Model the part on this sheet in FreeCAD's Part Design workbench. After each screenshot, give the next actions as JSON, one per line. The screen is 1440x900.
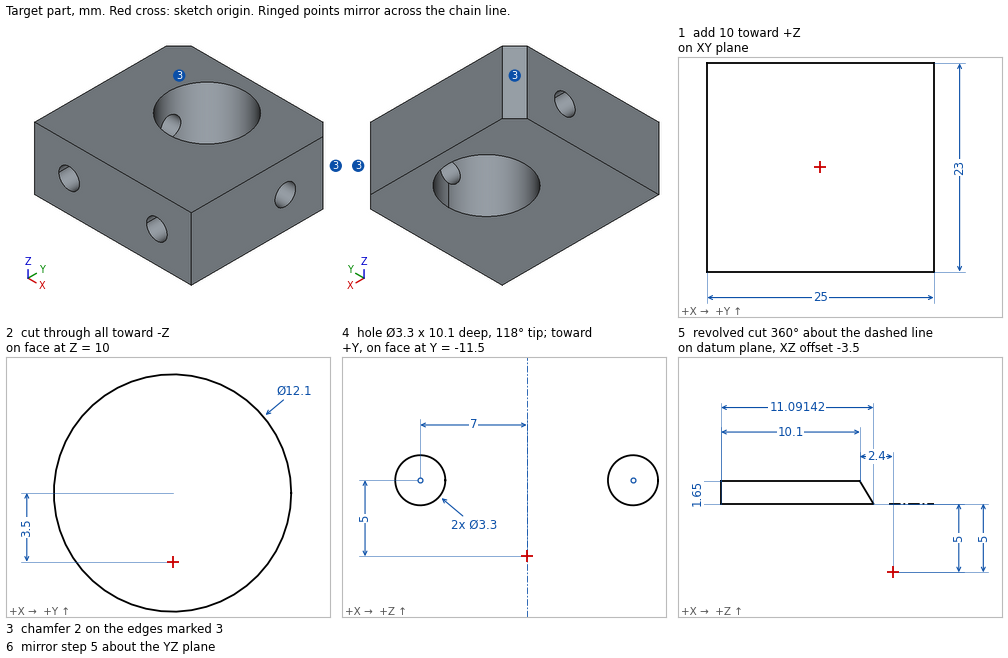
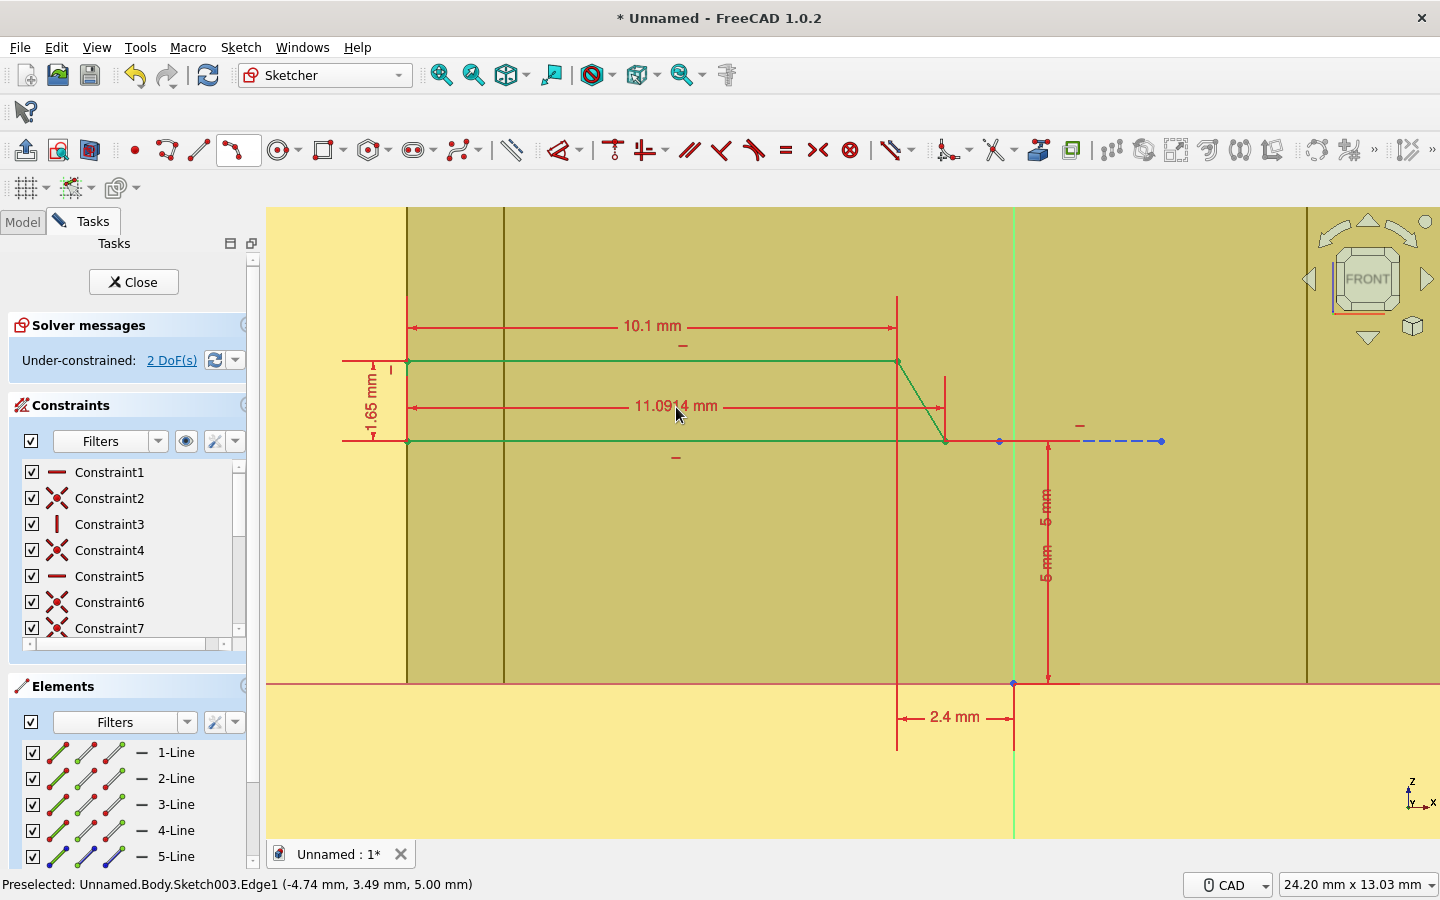
{"action": "left_click", "coordinate": [134, 282]}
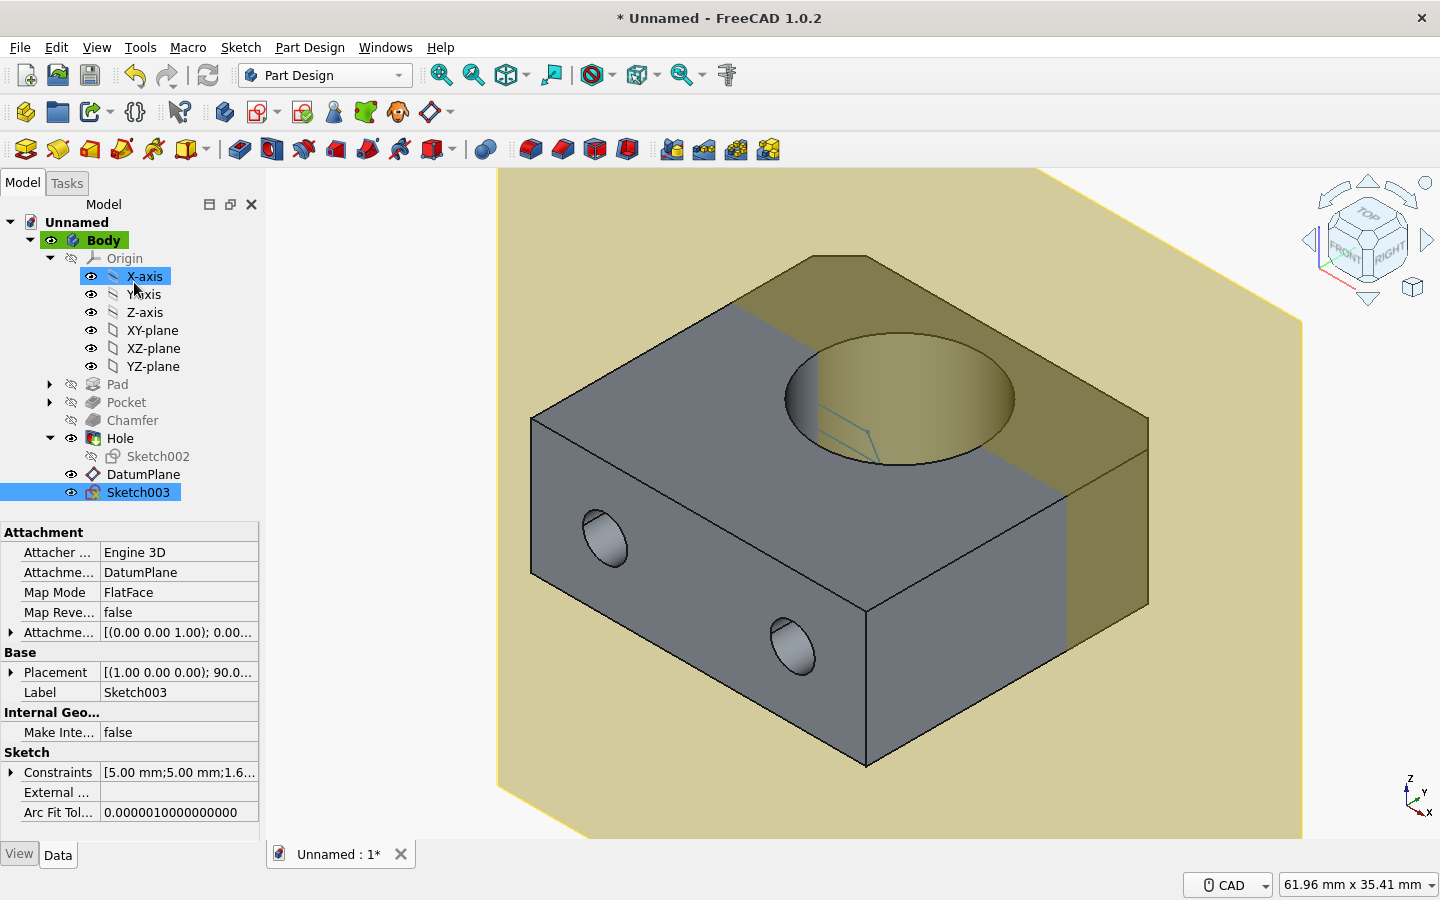
{"action": "left_click", "coordinate": [304, 150]}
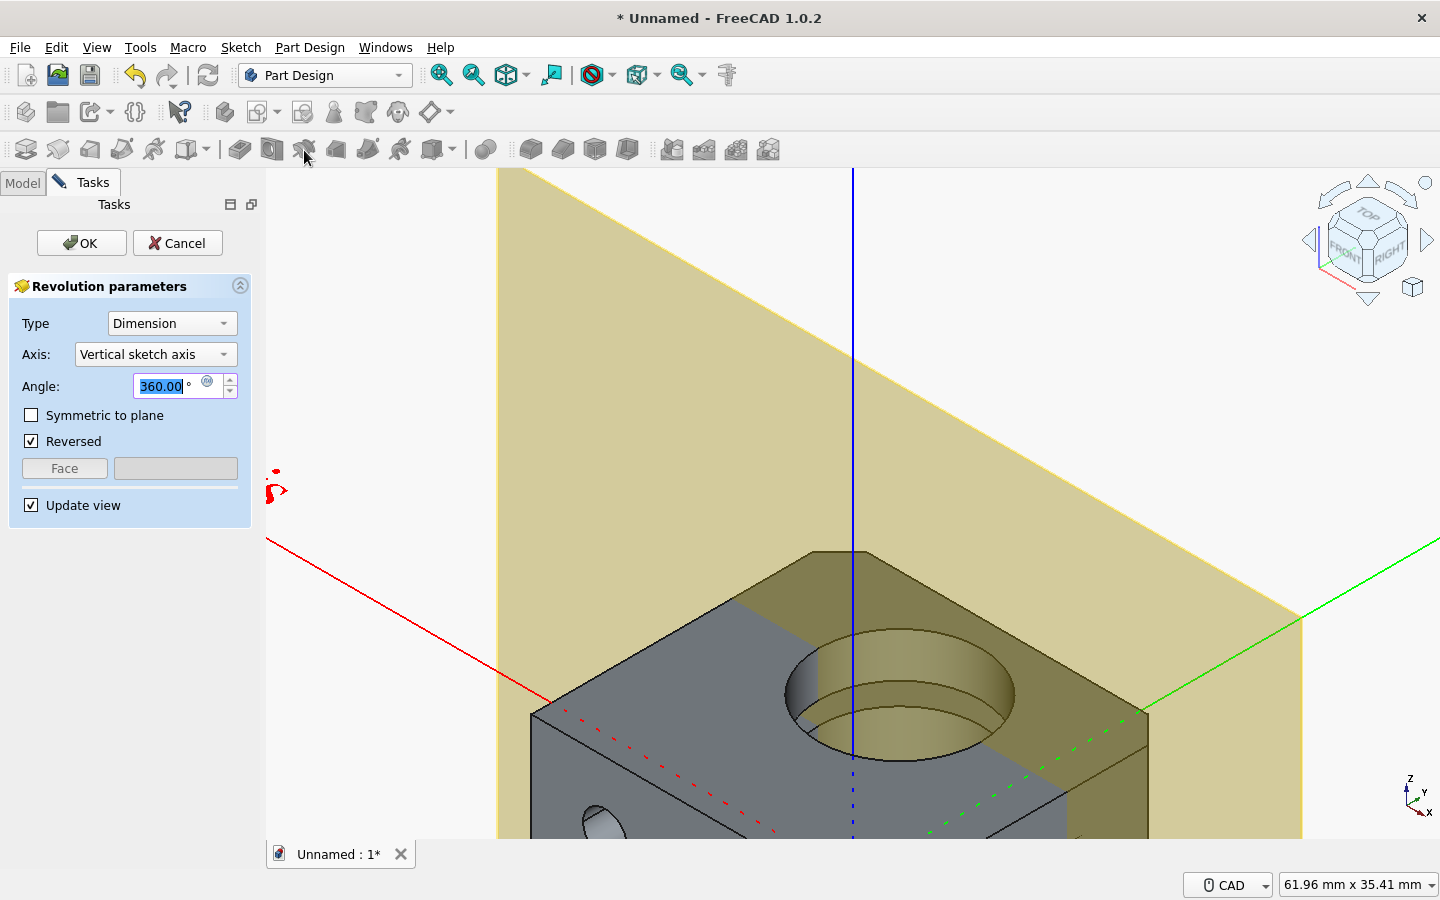
{"action": "left_click", "coordinate": [156, 354]}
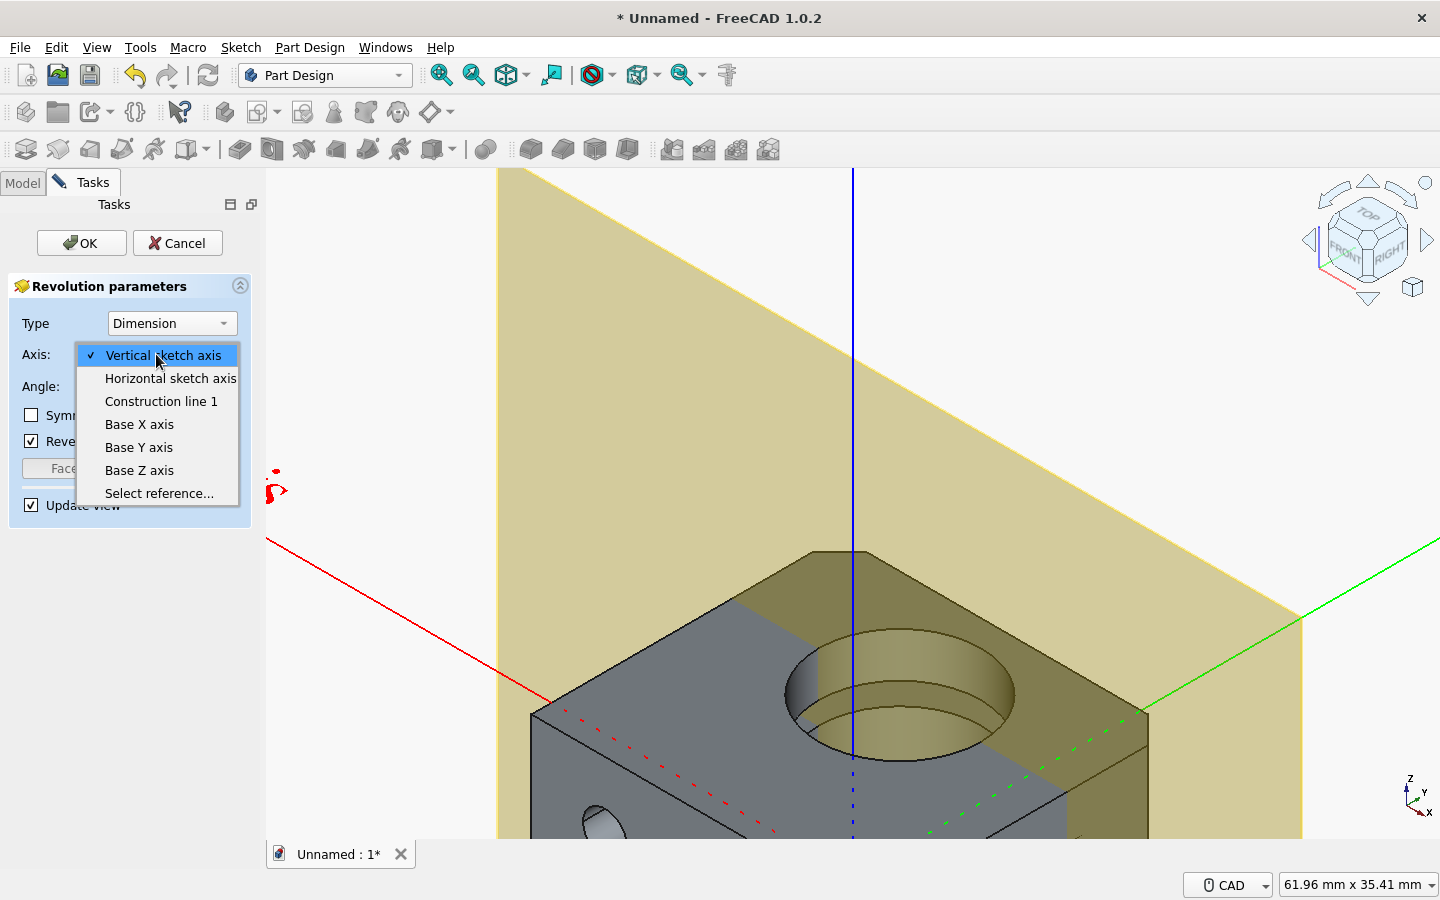
{"action": "left_click", "coordinate": [156, 402]}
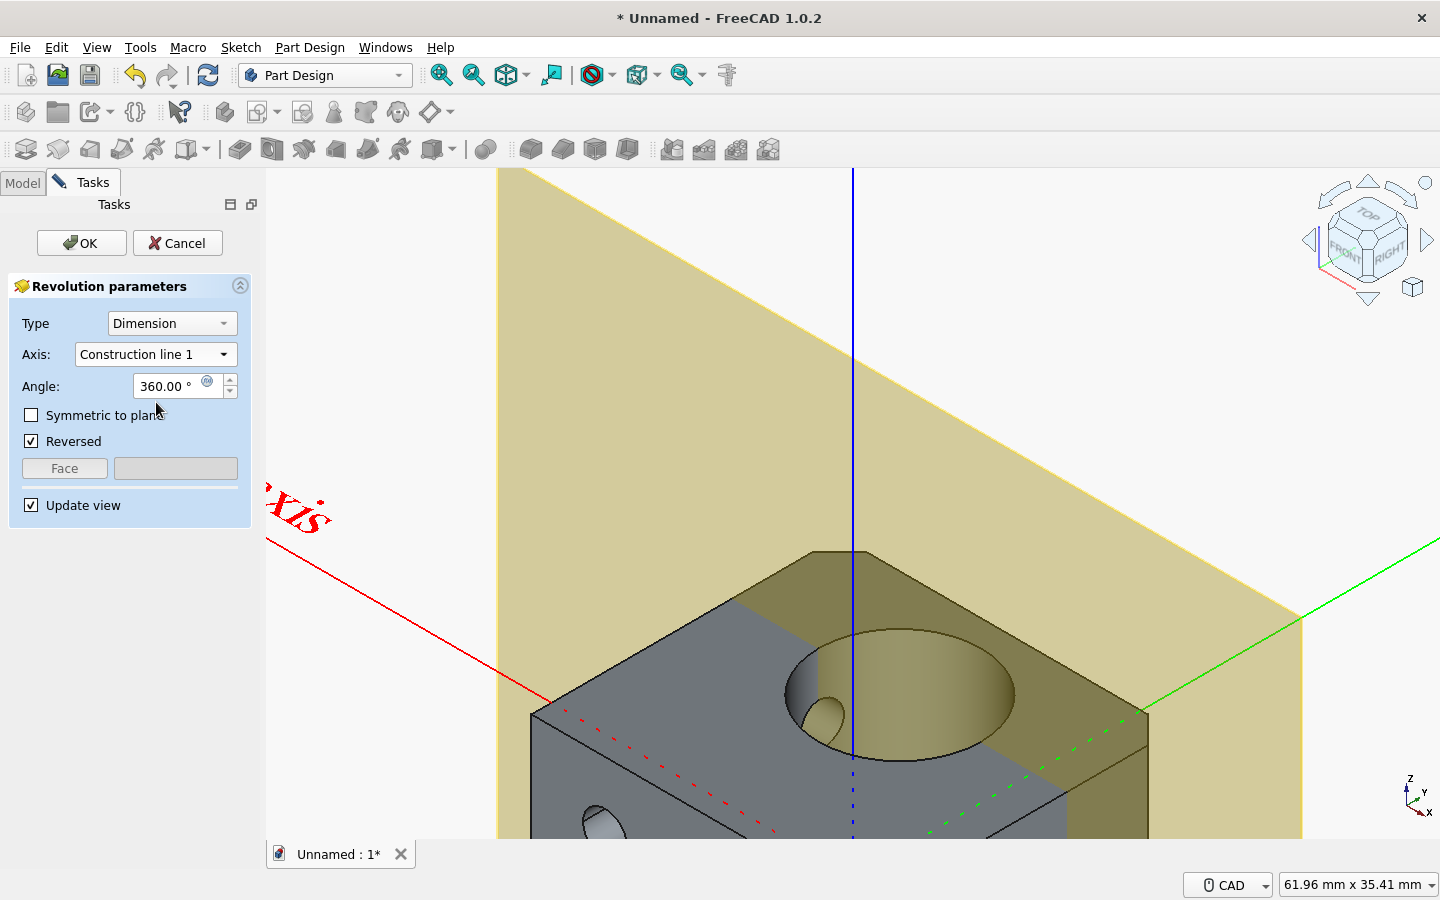
{"action": "left_click", "coordinate": [82, 243]}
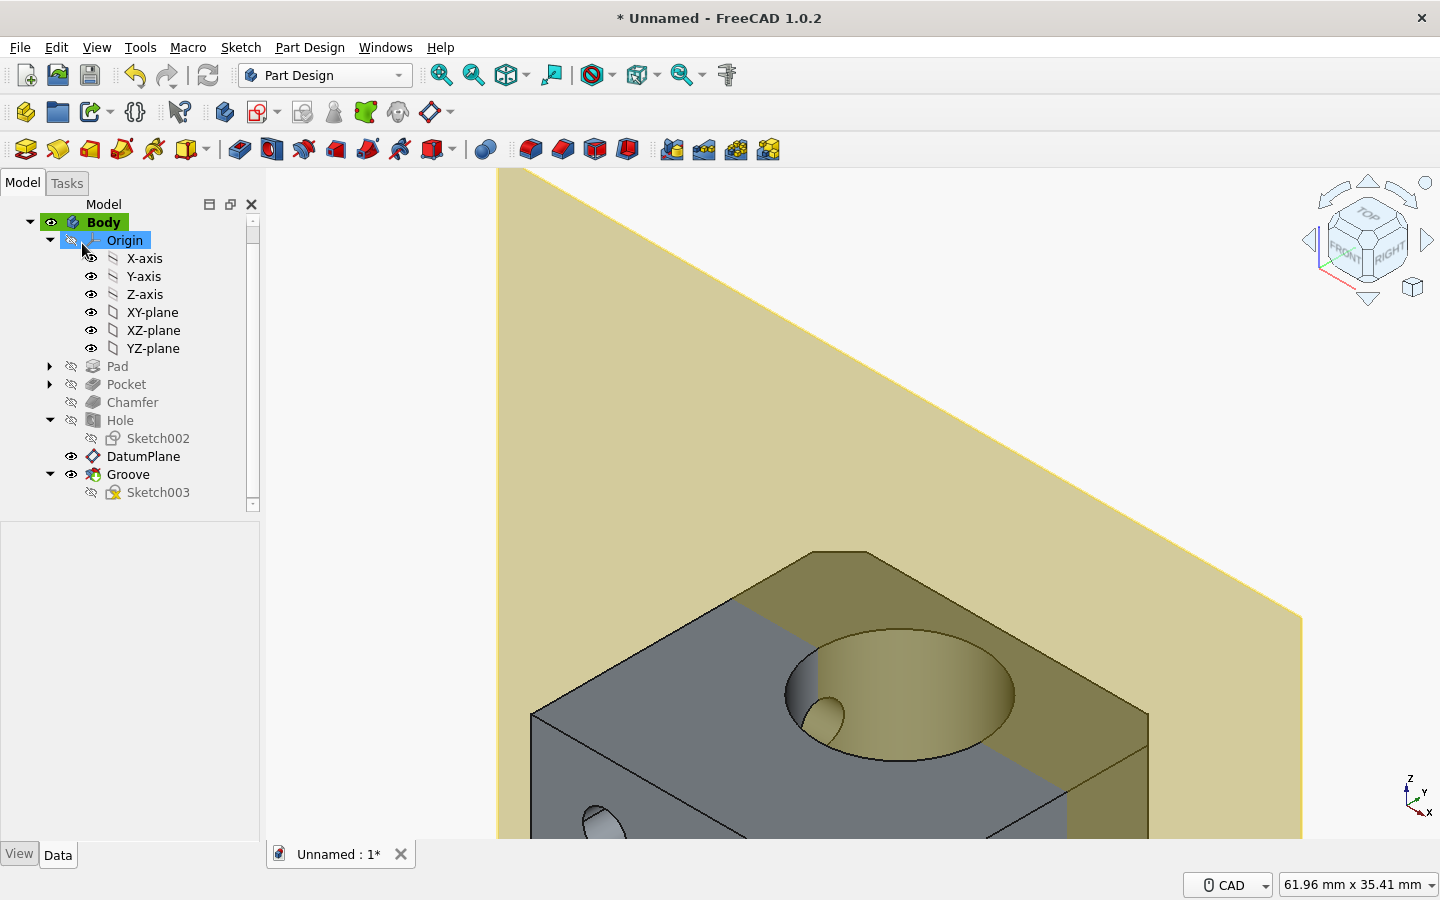
{"action": "left_click", "coordinate": [116, 456]}
{"action": "key", "text": "space"}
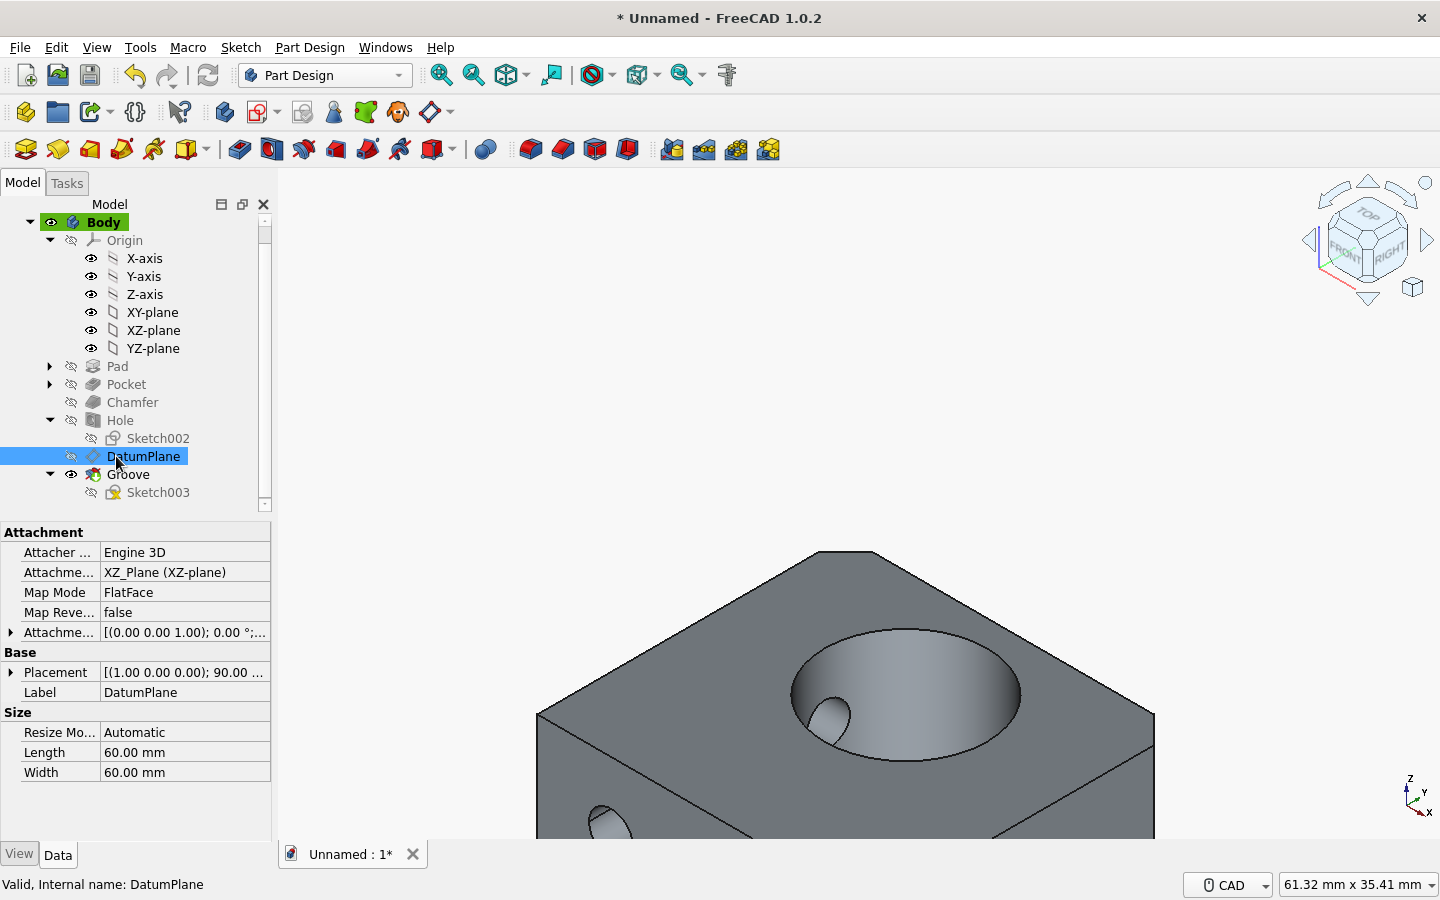
{"action": "left_click", "coordinate": [442, 76]}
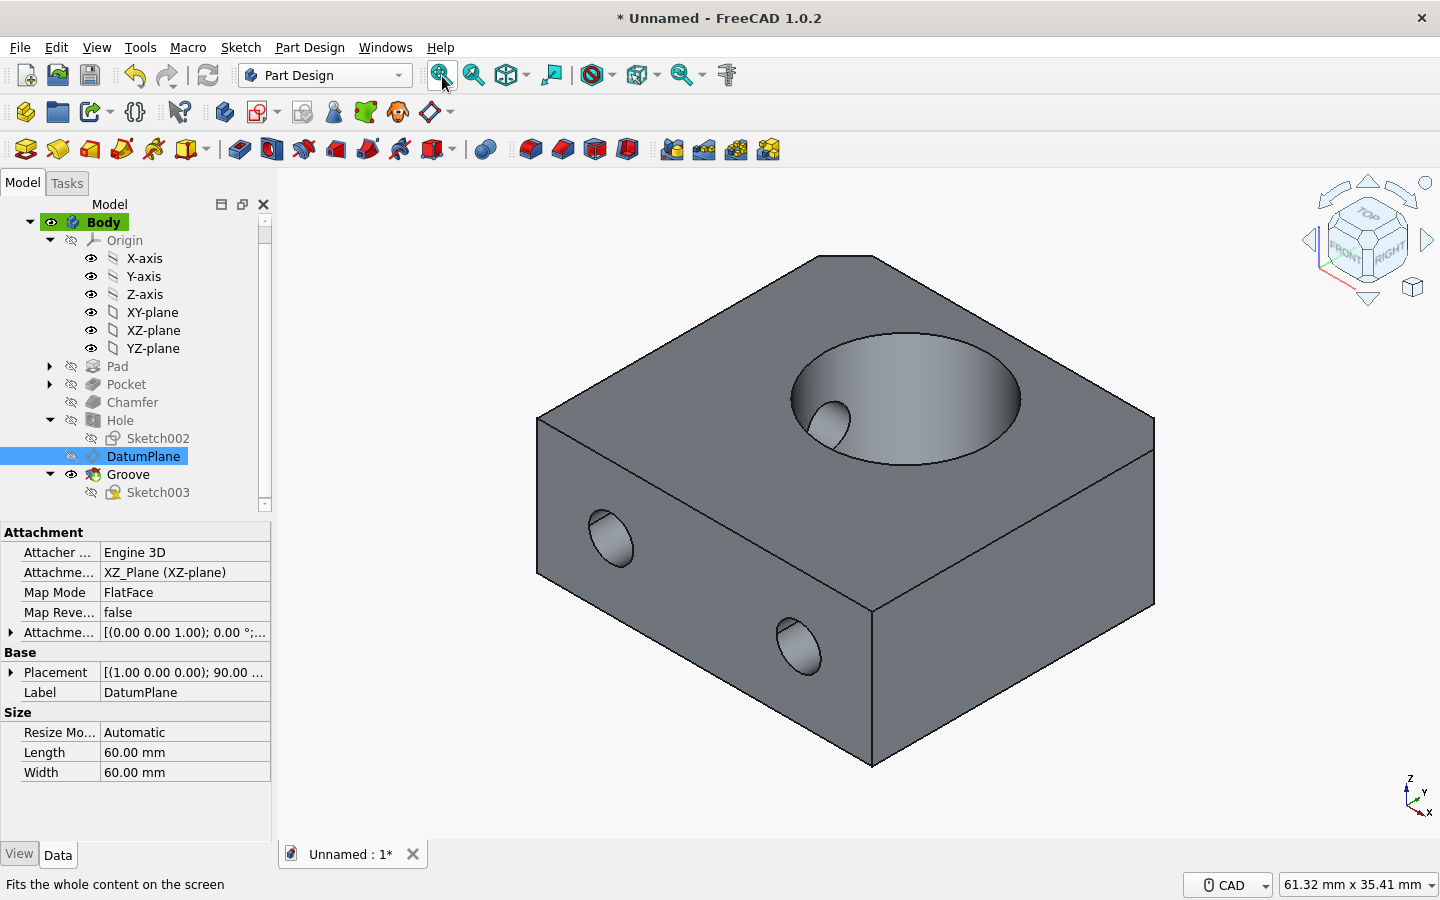
{"action": "left_click", "coordinate": [116, 474]}